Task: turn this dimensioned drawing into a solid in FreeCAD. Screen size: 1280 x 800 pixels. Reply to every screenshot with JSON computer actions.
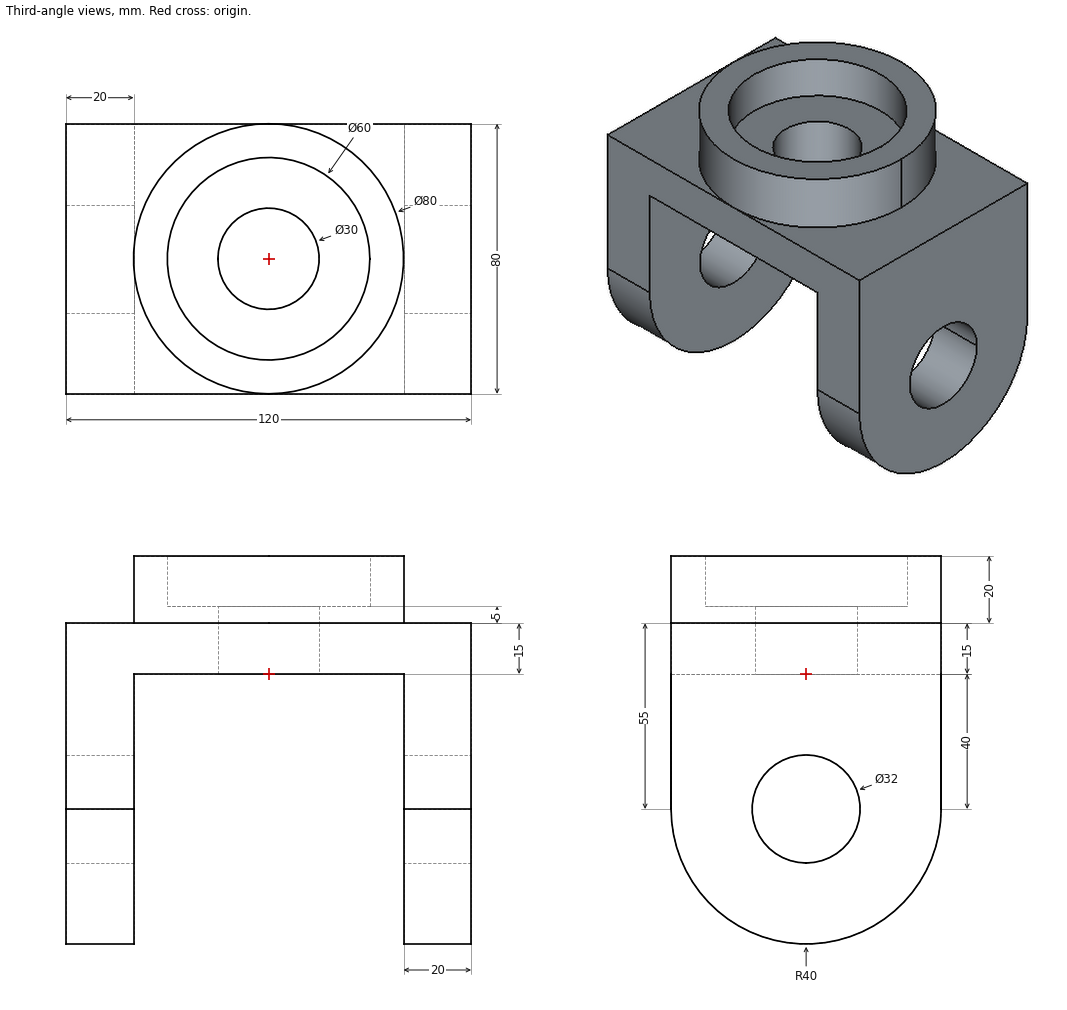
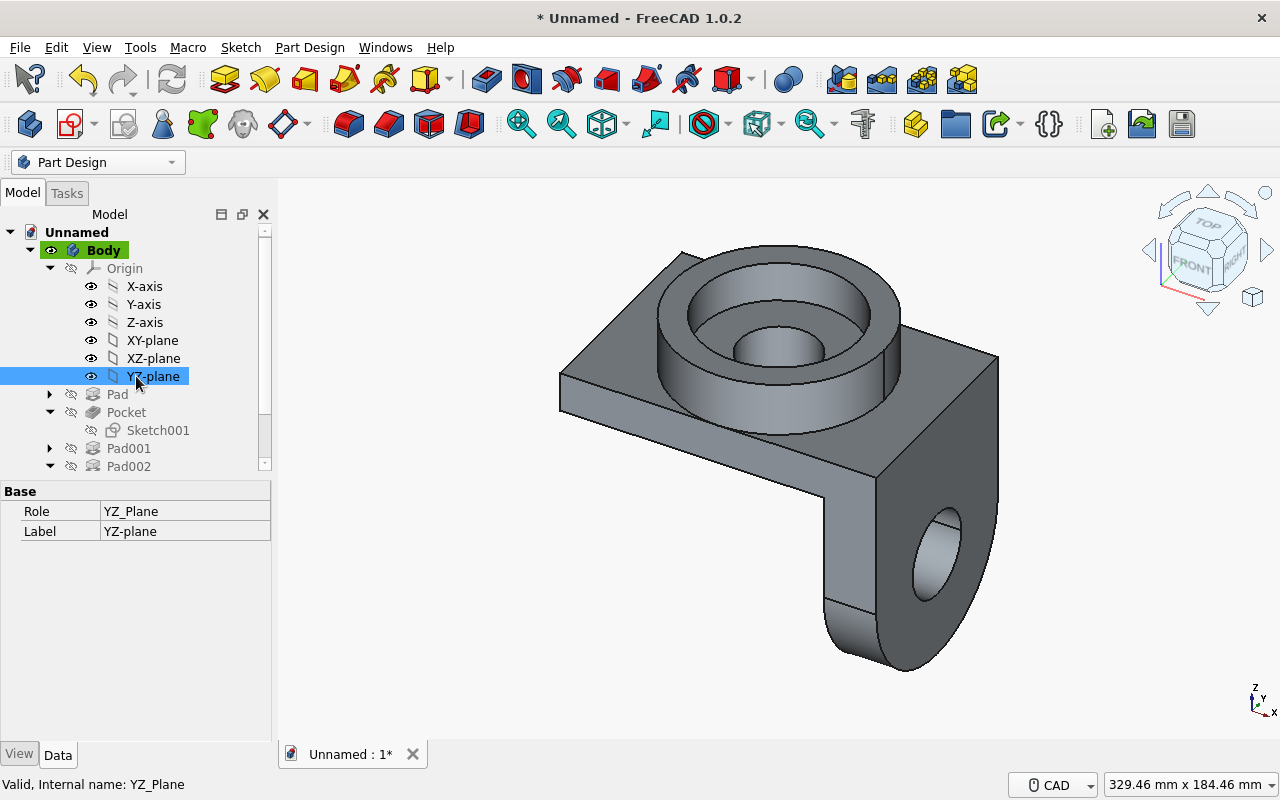
{"action": "left_click", "coordinate": [284, 124]}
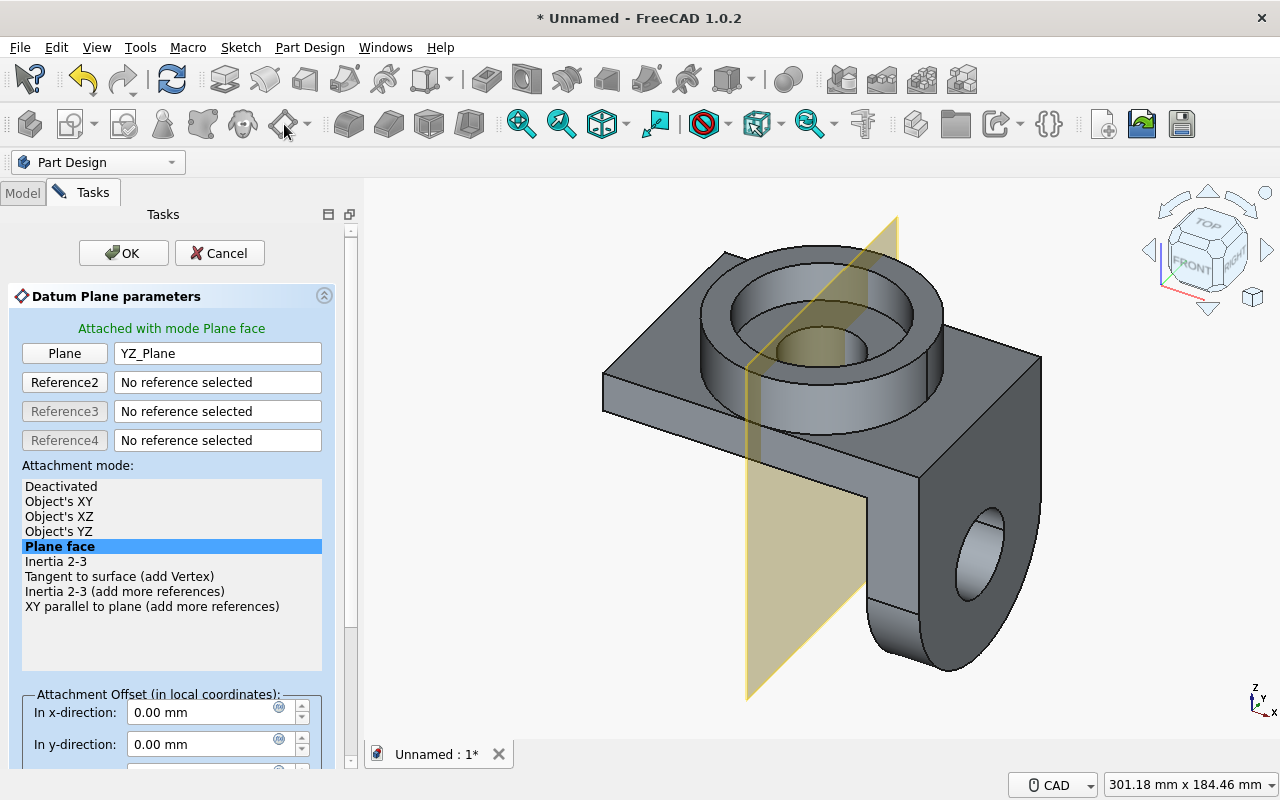
{"action": "scroll", "coordinate": [351, 496], "scroll_direction": "down", "scroll_amount": 2}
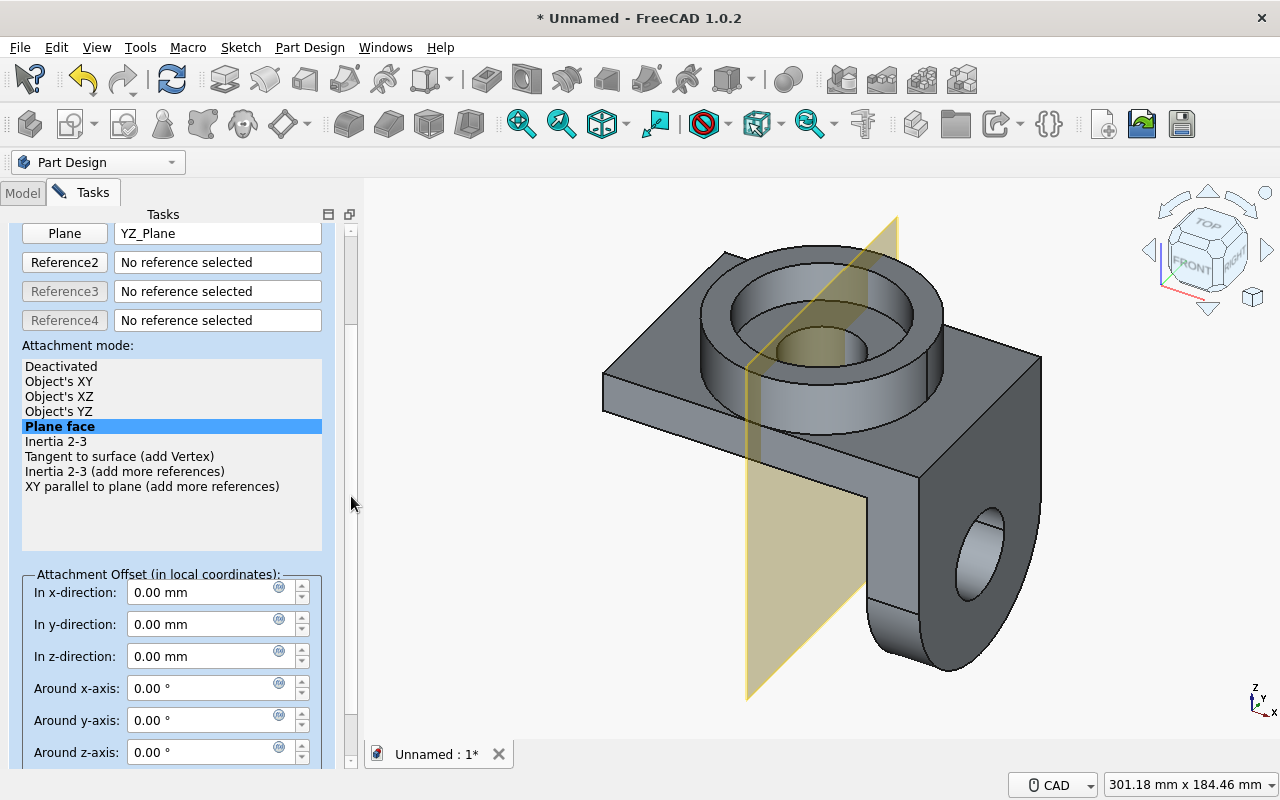
{"action": "triple_click", "coordinate": [210, 656]}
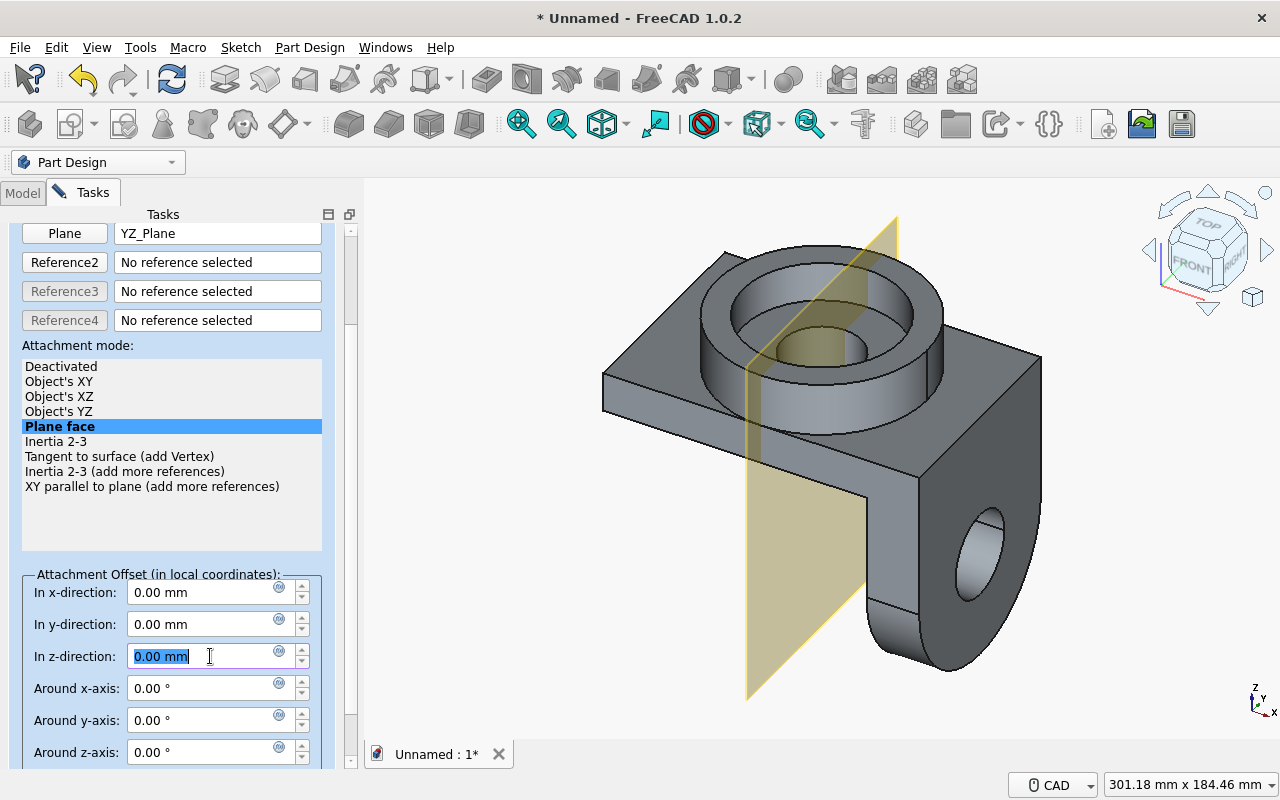
{"action": "type", "text": "-40"}
{"action": "key", "text": "Tab"}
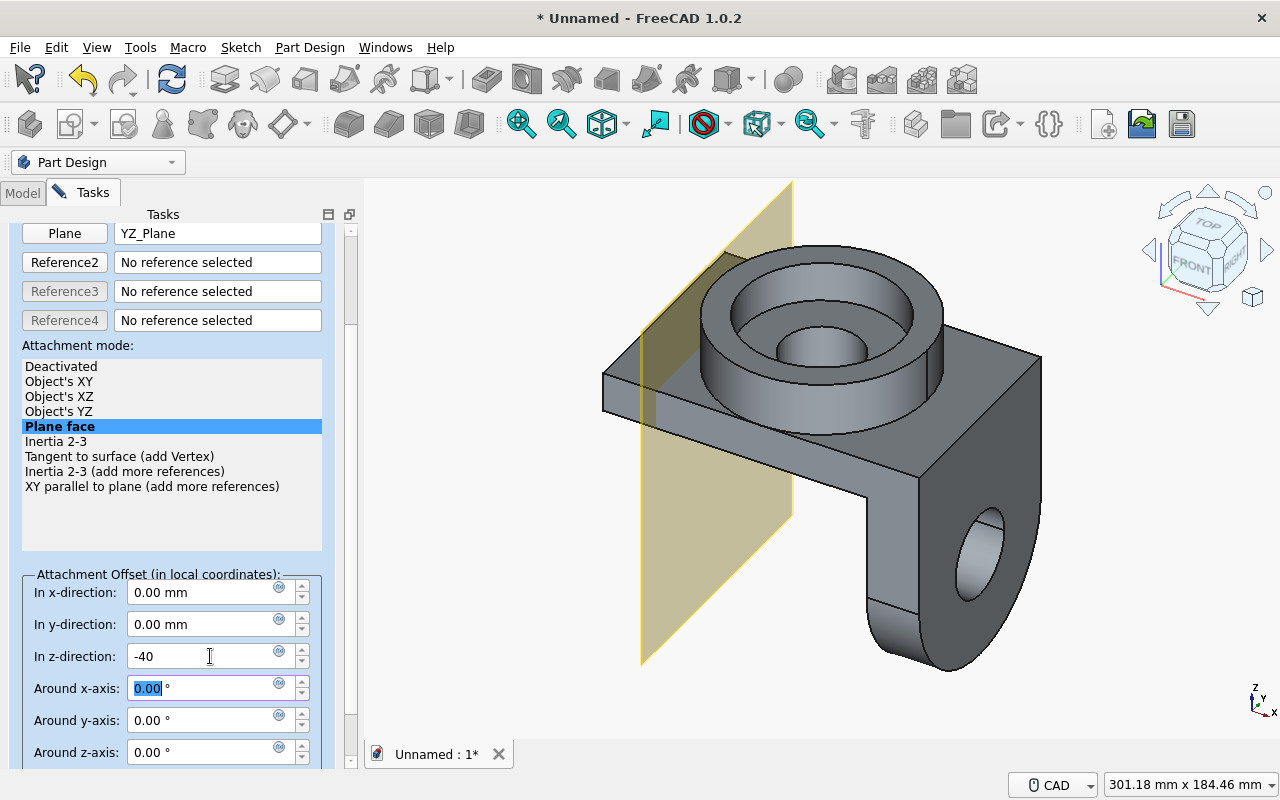
{"action": "scroll", "coordinate": [351, 496], "scroll_direction": "up", "scroll_amount": 3}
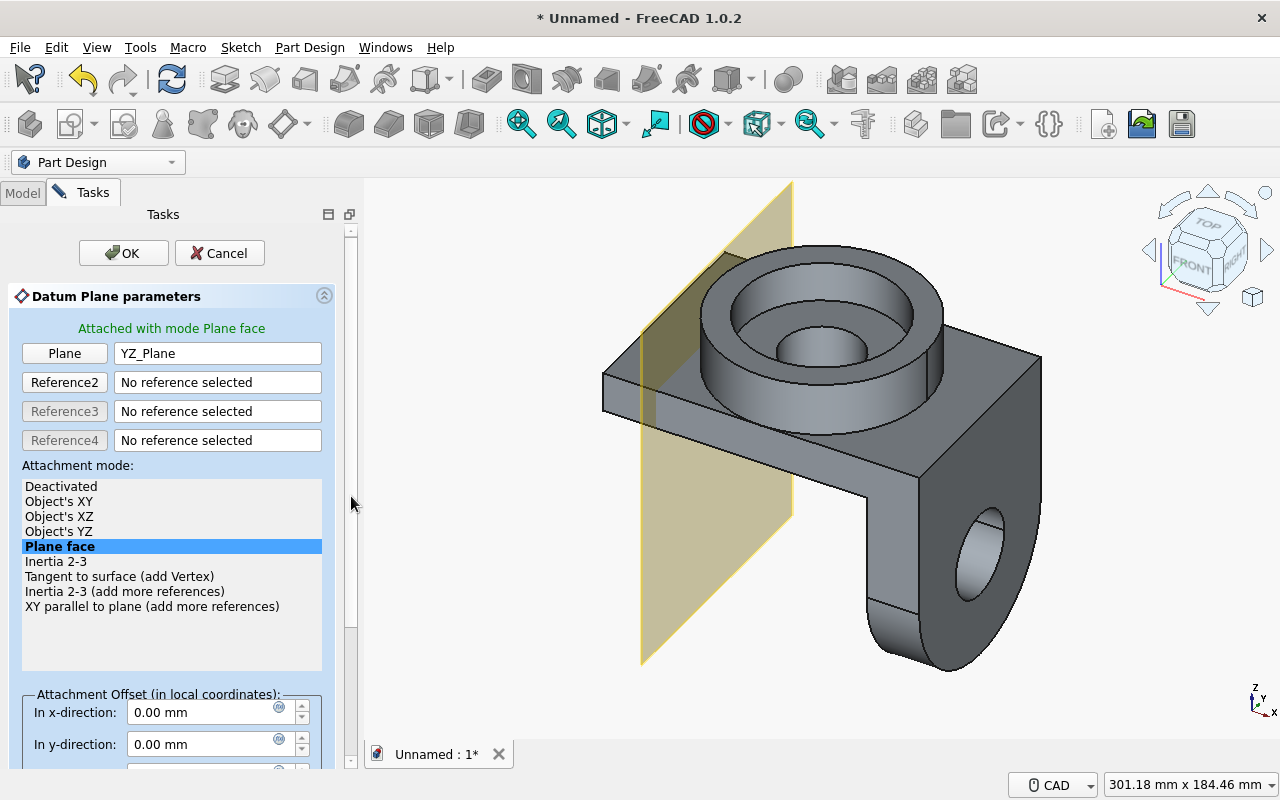
{"action": "left_click", "coordinate": [124, 253]}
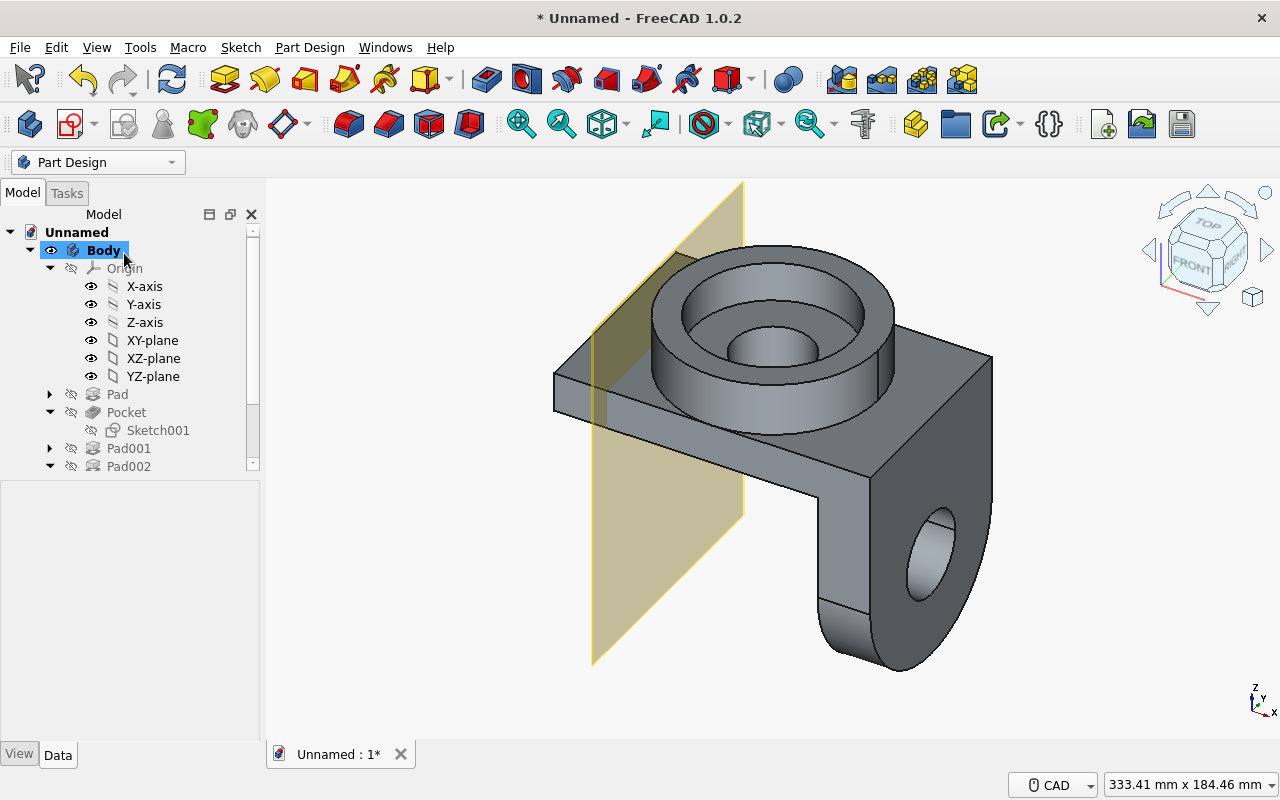
{"action": "scroll", "coordinate": [100, 354], "scroll_direction": "down", "scroll_amount": 3}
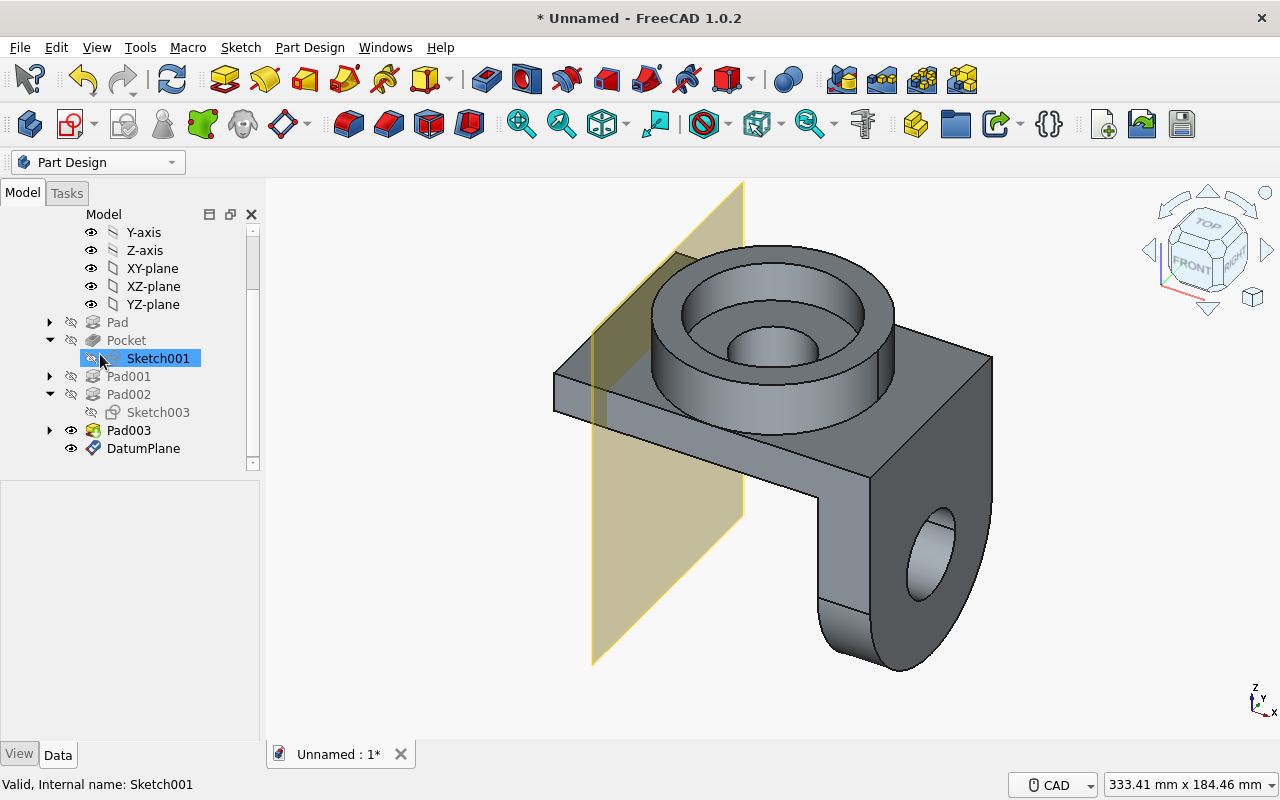
{"action": "left_click", "coordinate": [116, 448]}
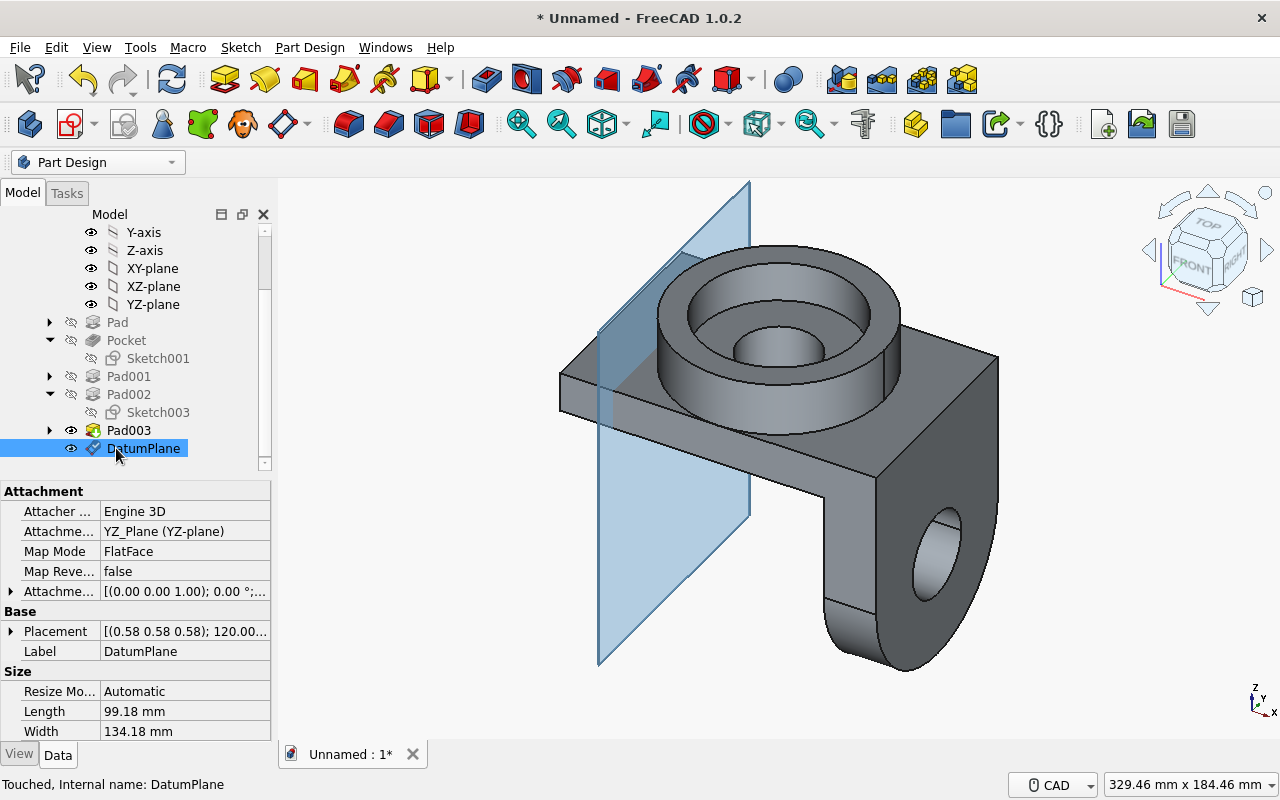
{"action": "left_click", "coordinate": [70, 124]}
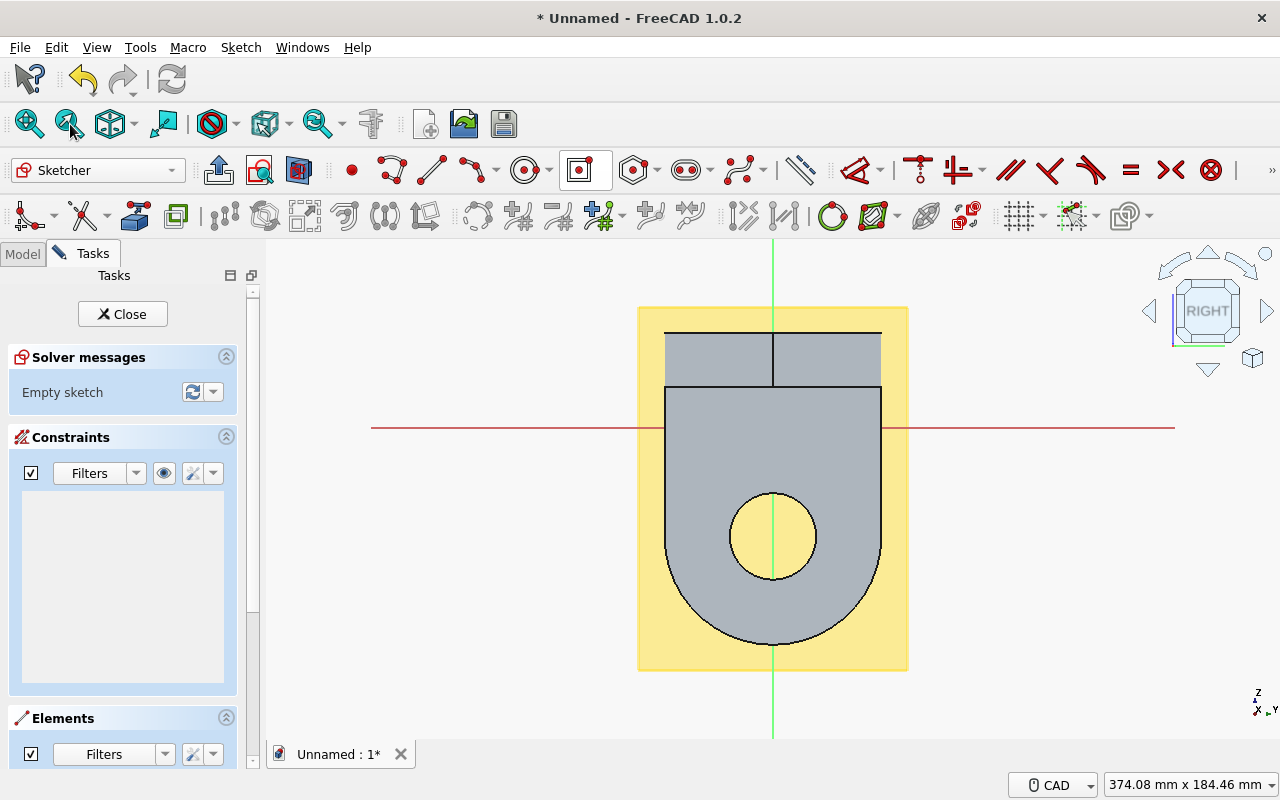
{"action": "left_click", "coordinate": [300, 170]}